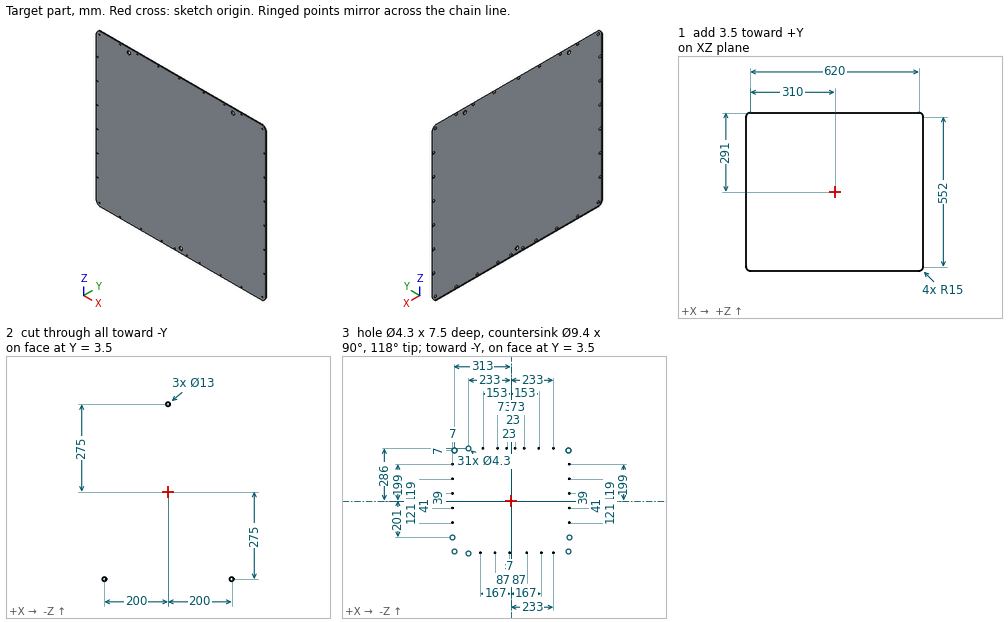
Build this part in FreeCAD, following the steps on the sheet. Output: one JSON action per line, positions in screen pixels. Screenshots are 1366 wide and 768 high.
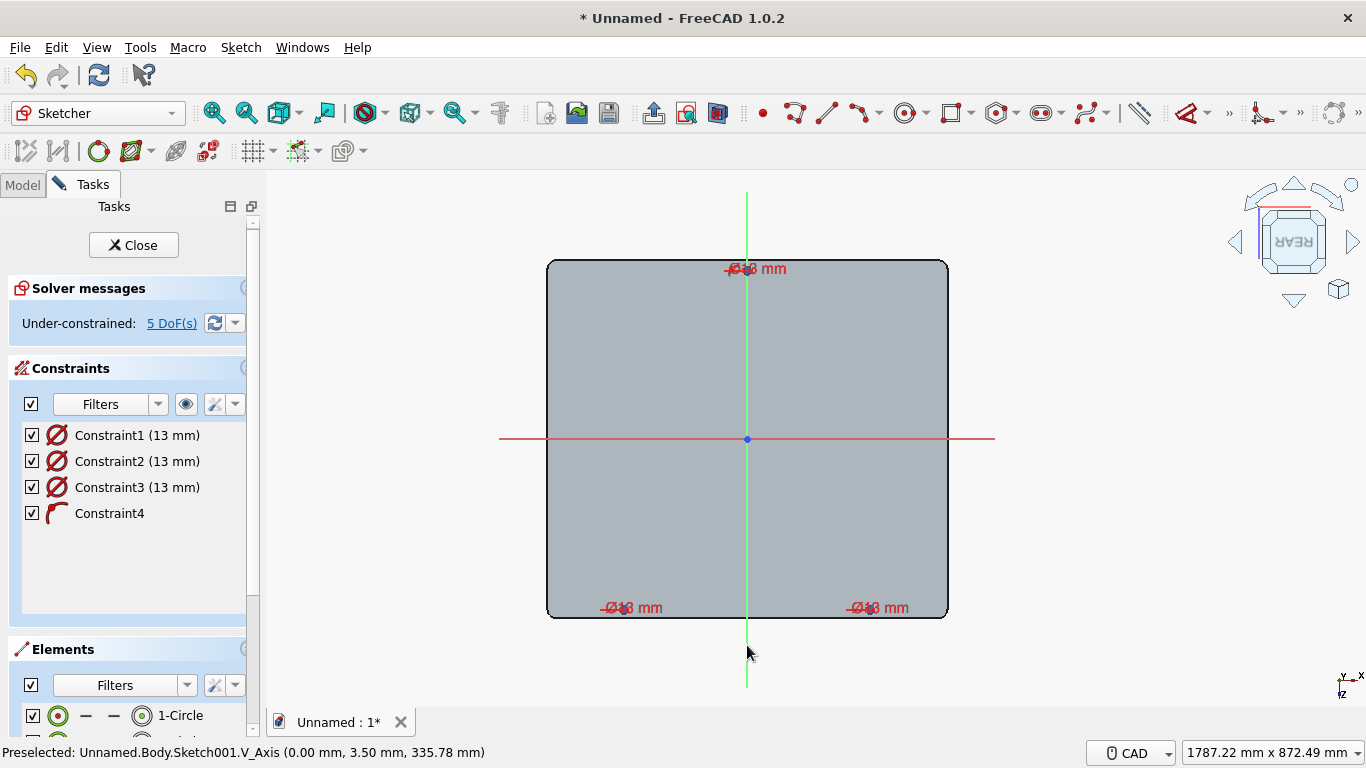
{"action": "left_click", "coordinate": [870, 610]}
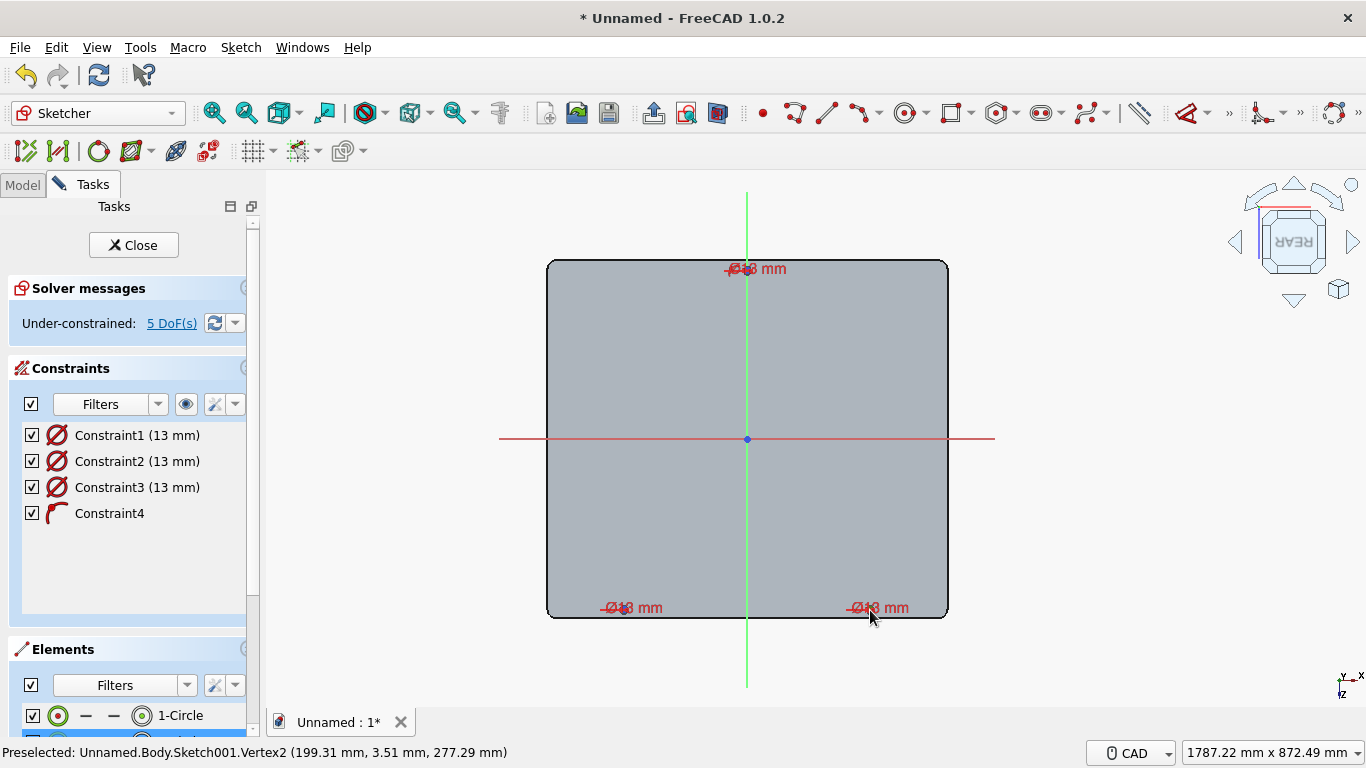
{"action": "left_click", "coordinate": [624, 610]}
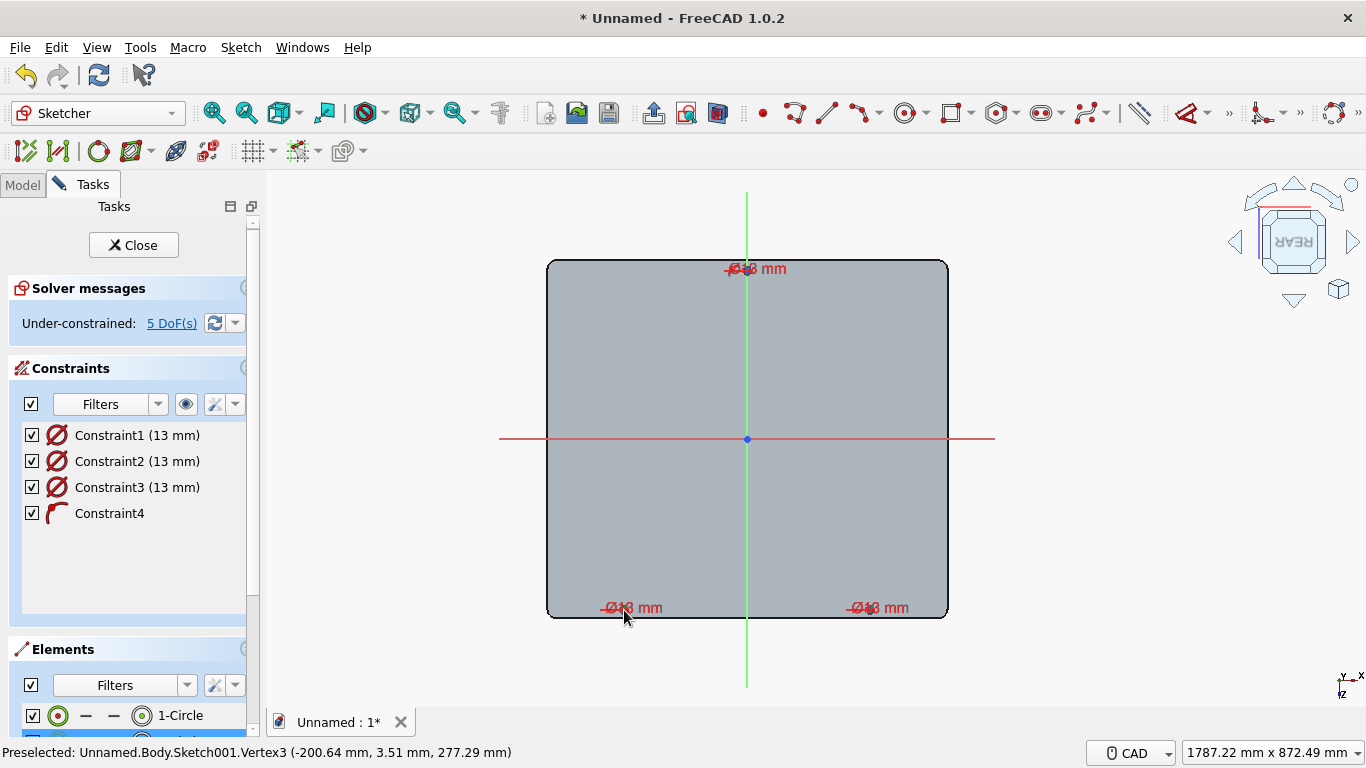
{"action": "key", "text": "h"}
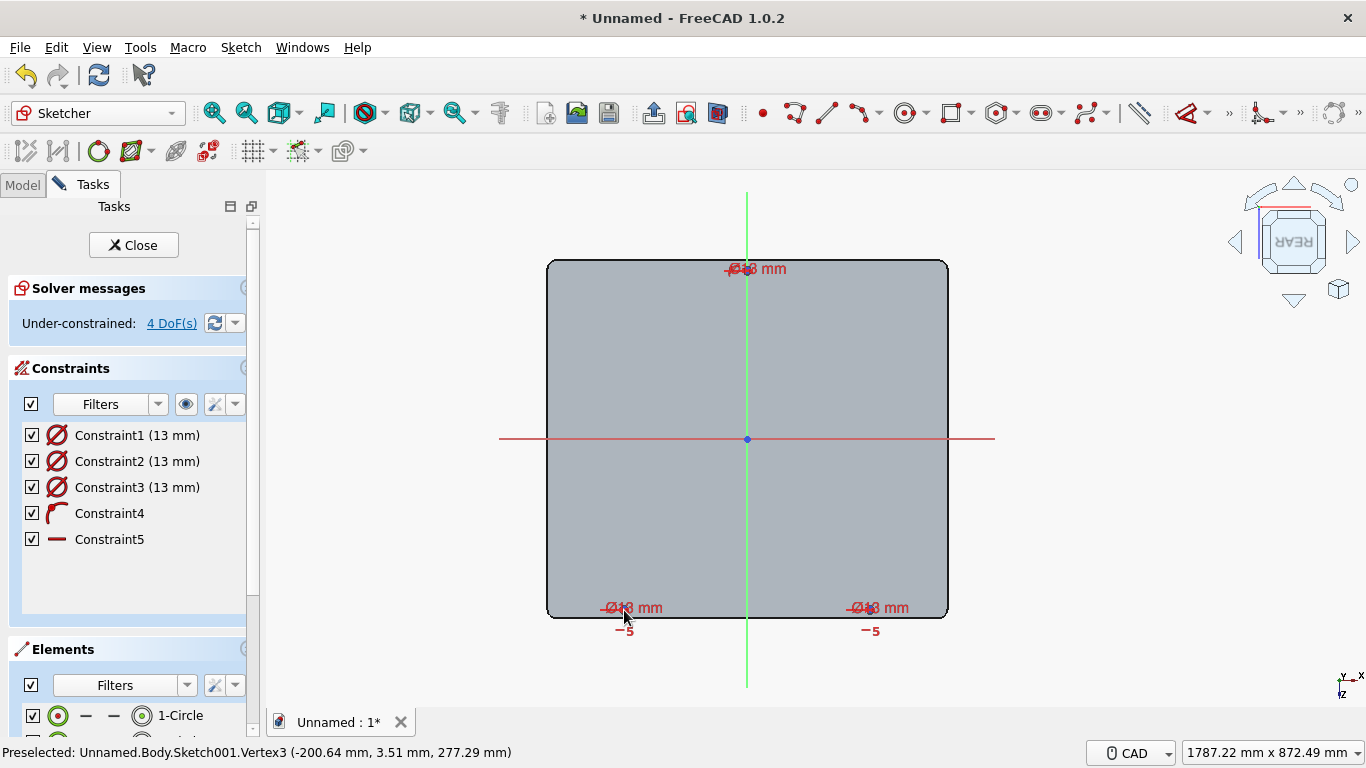
{"action": "left_click", "coordinate": [1186, 114]}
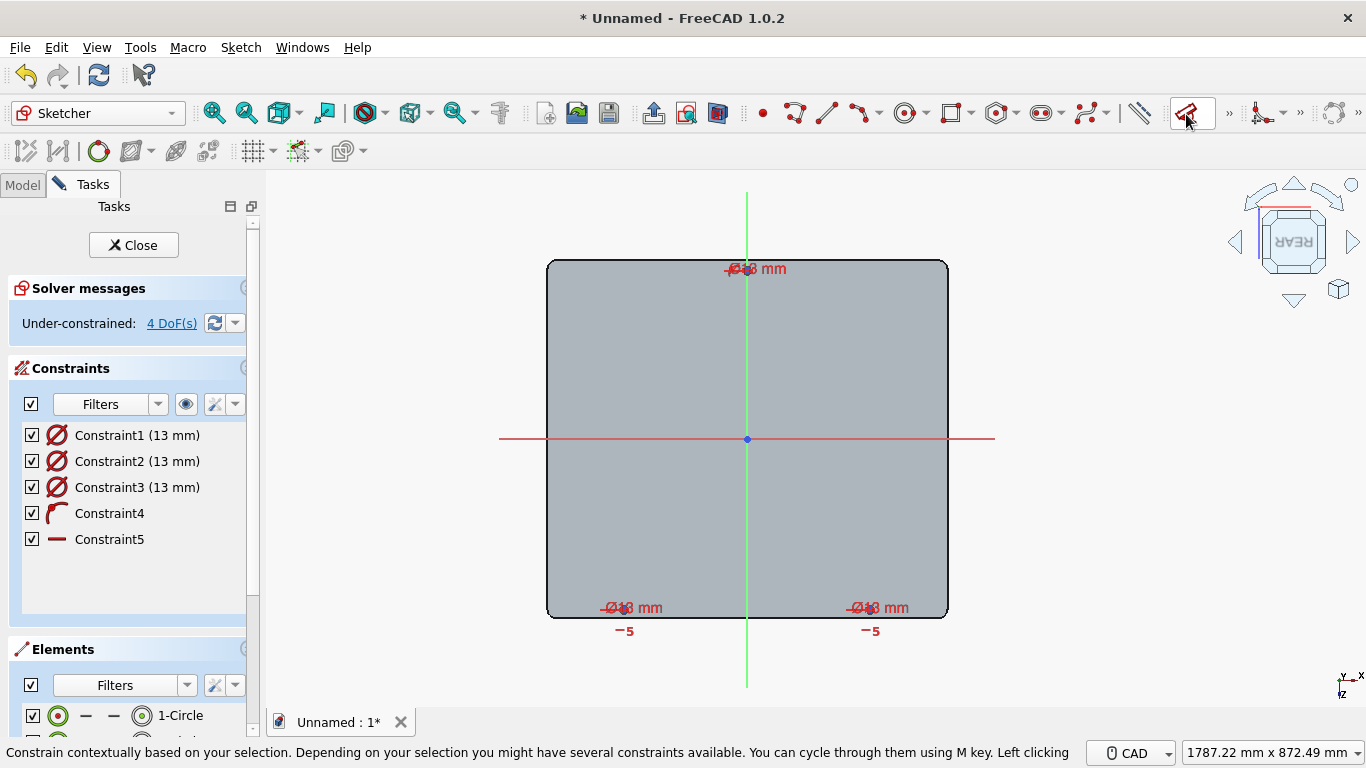
{"action": "left_click", "coordinate": [747, 271]}
{"action": "left_click", "coordinate": [781, 355]}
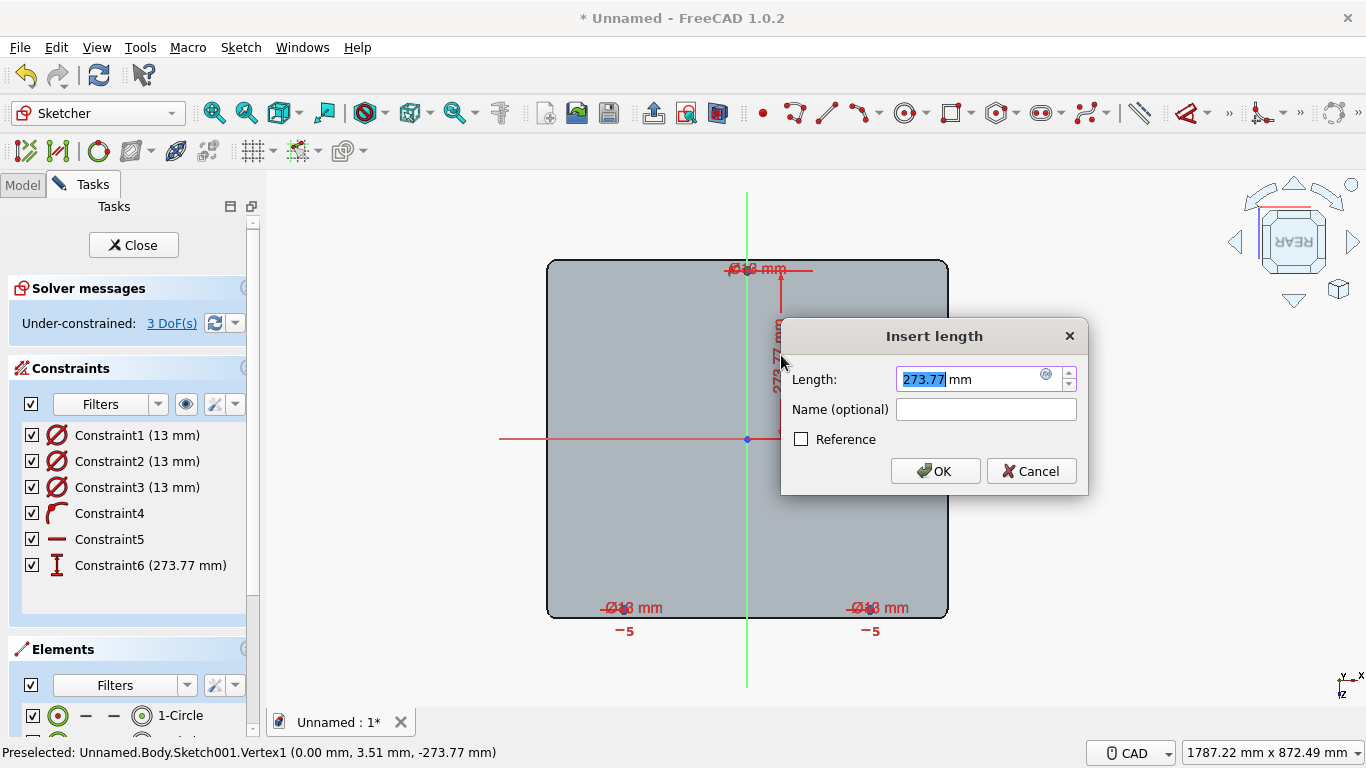
{"action": "type", "text": "275"}
{"action": "key", "text": "Return"}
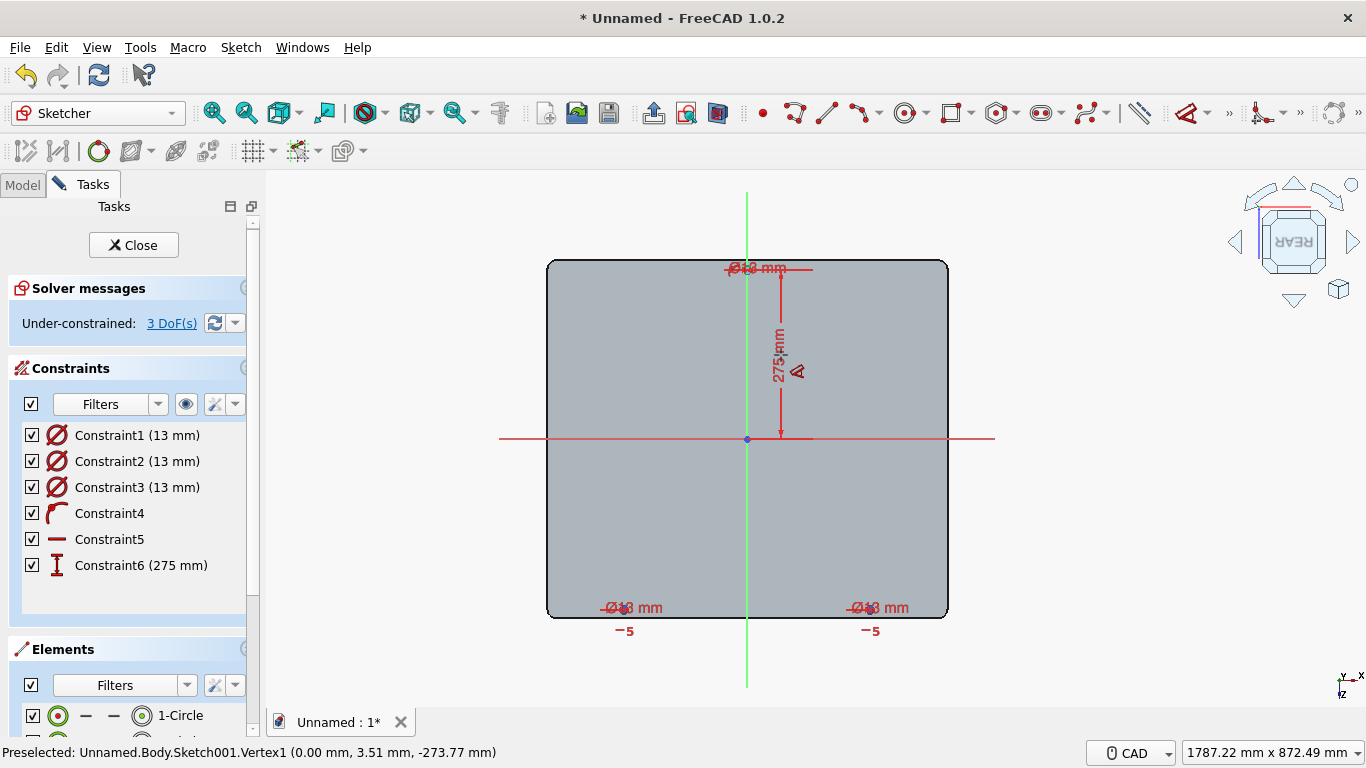
{"action": "left_click", "coordinate": [870, 610]}
{"action": "left_click", "coordinate": [809, 644]}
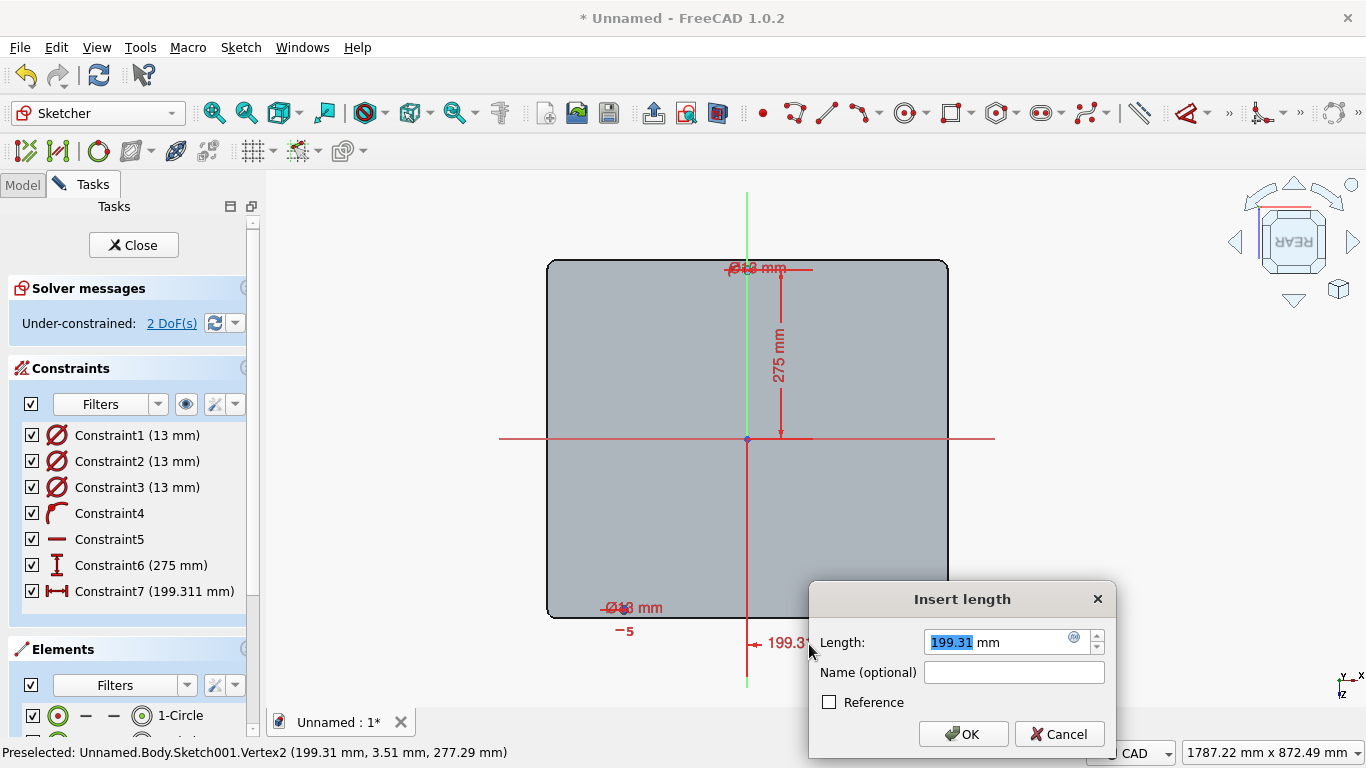
{"action": "type", "text": "200"}
{"action": "key", "text": "Return"}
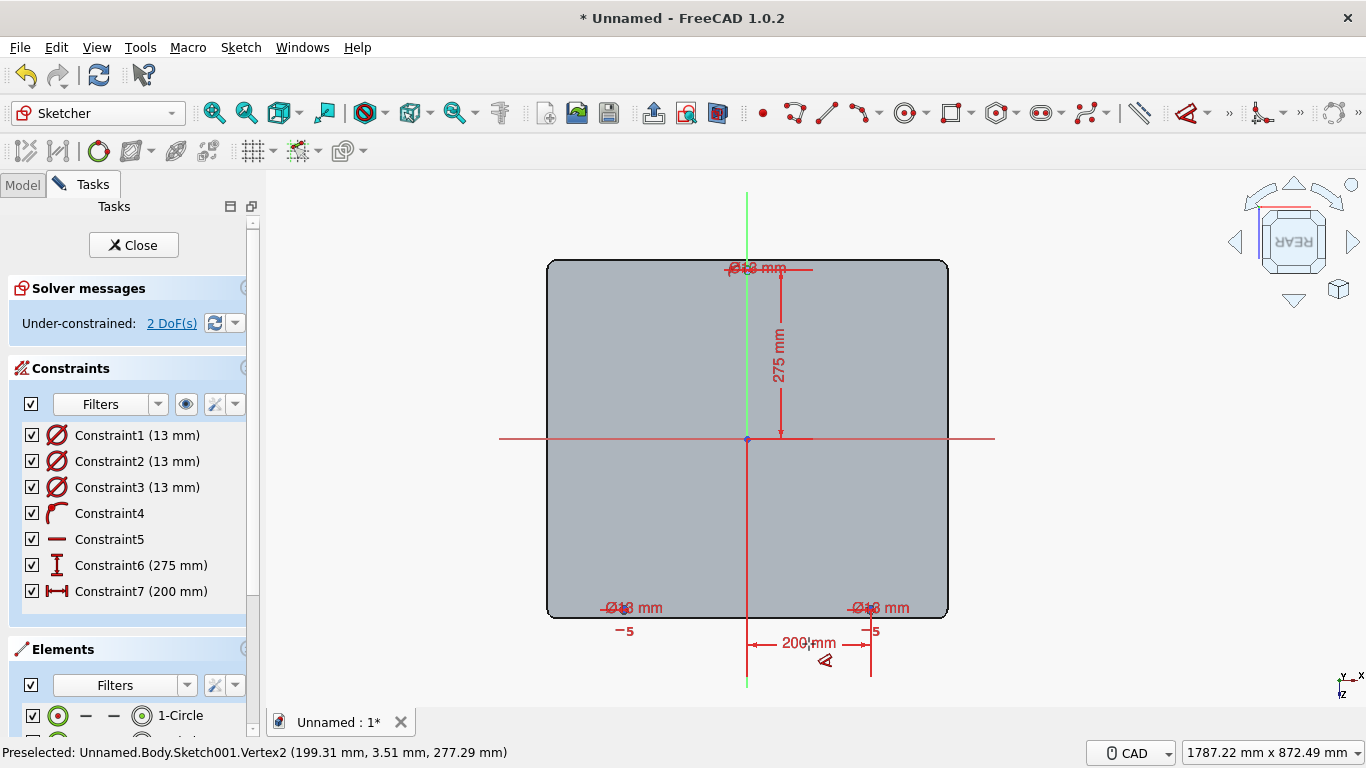
{"action": "left_click", "coordinate": [871, 610]}
{"action": "left_click", "coordinate": [905, 525]}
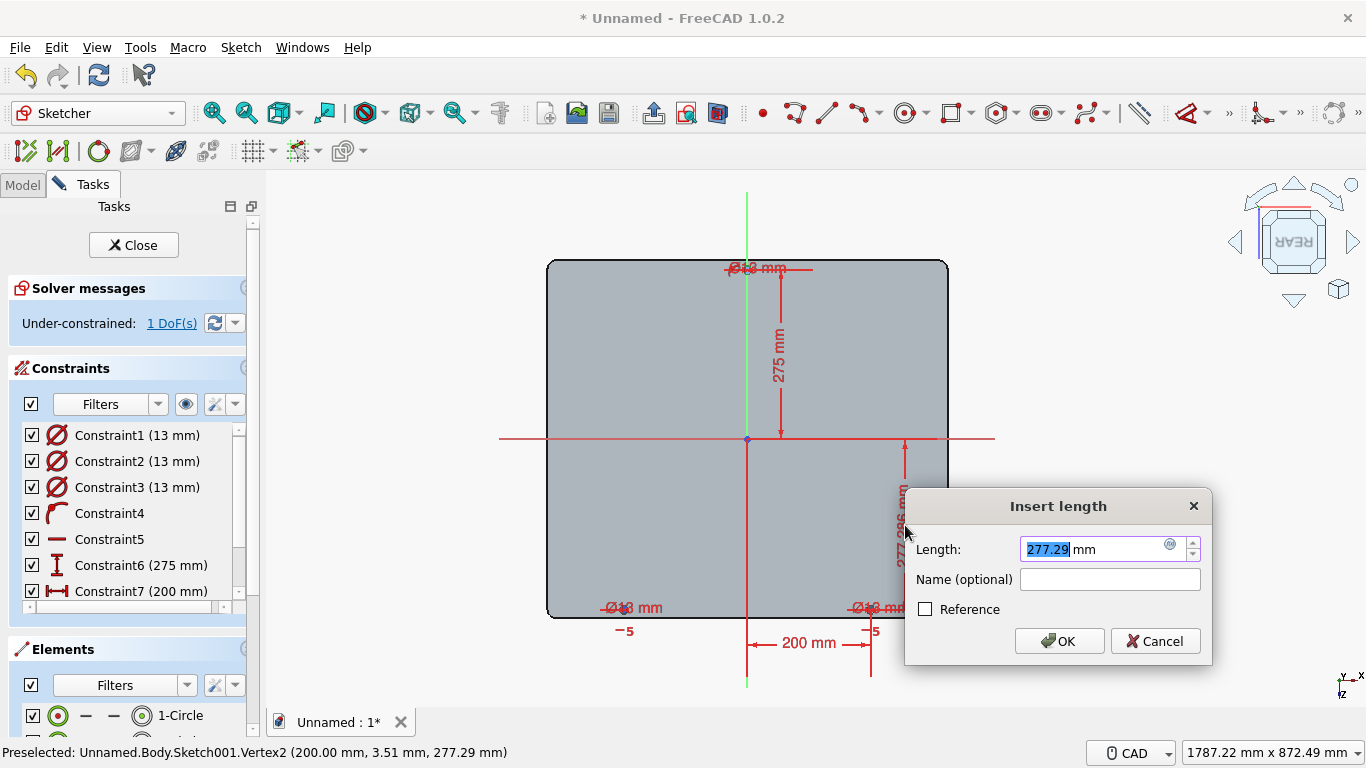
{"action": "type", "text": "275"}
{"action": "key", "text": "Return"}